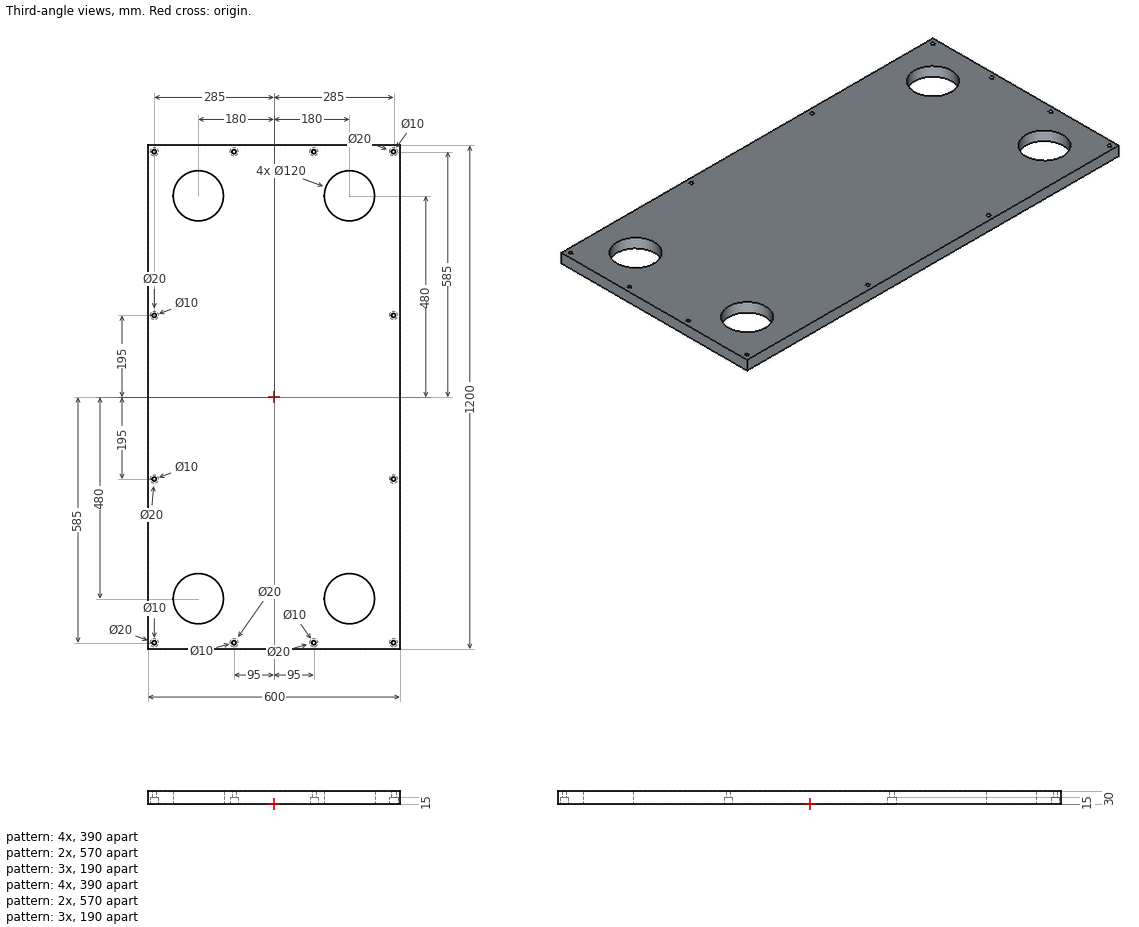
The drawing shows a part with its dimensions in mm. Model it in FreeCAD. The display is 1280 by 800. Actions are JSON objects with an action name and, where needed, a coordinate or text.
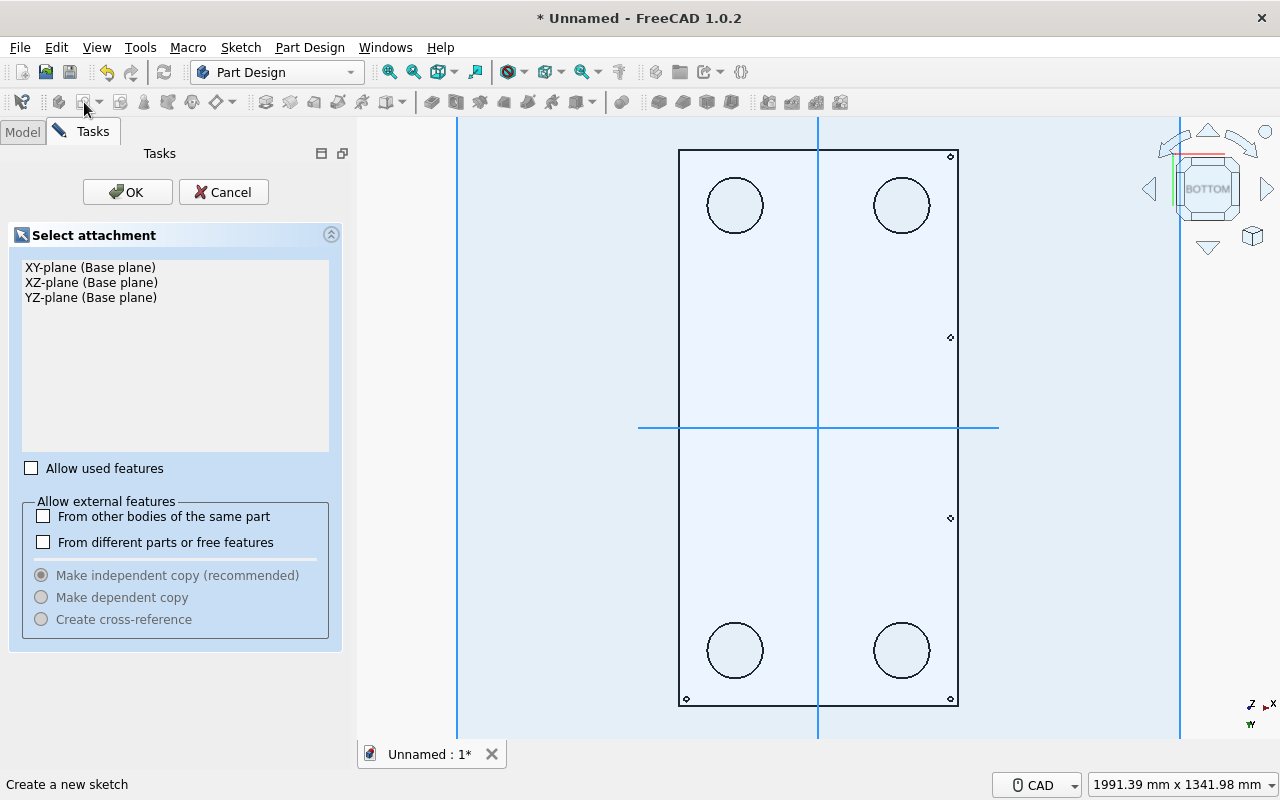
{"action": "left_click", "coordinate": [82, 268]}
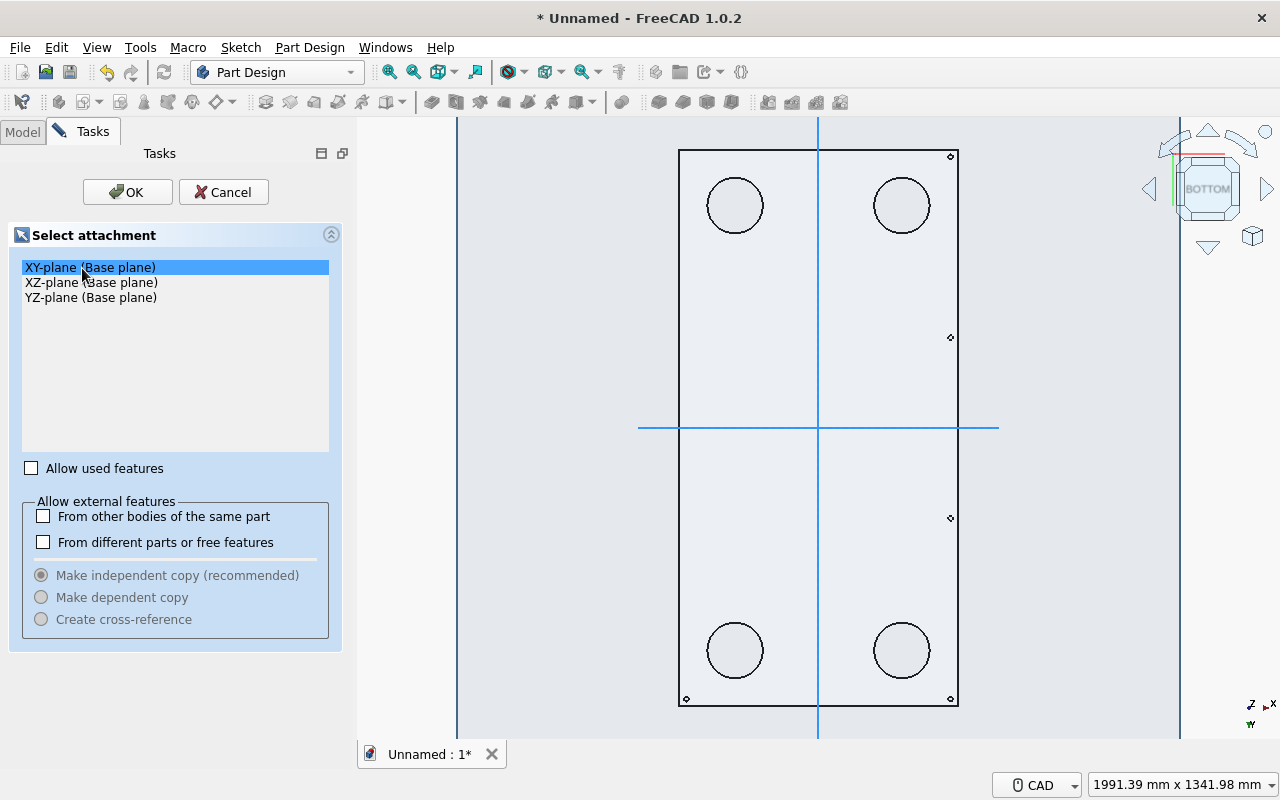
{"action": "left_click", "coordinate": [128, 192]}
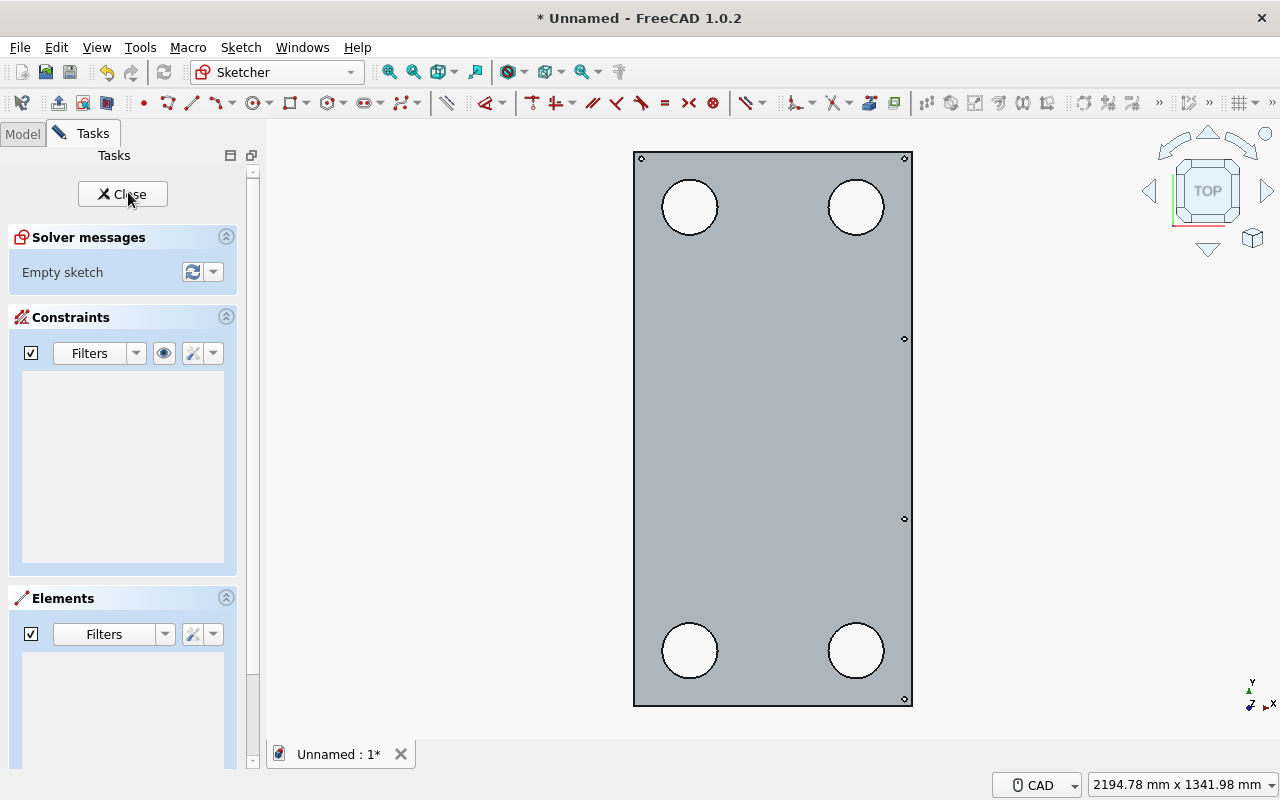
{"action": "left_click", "coordinate": [108, 104]}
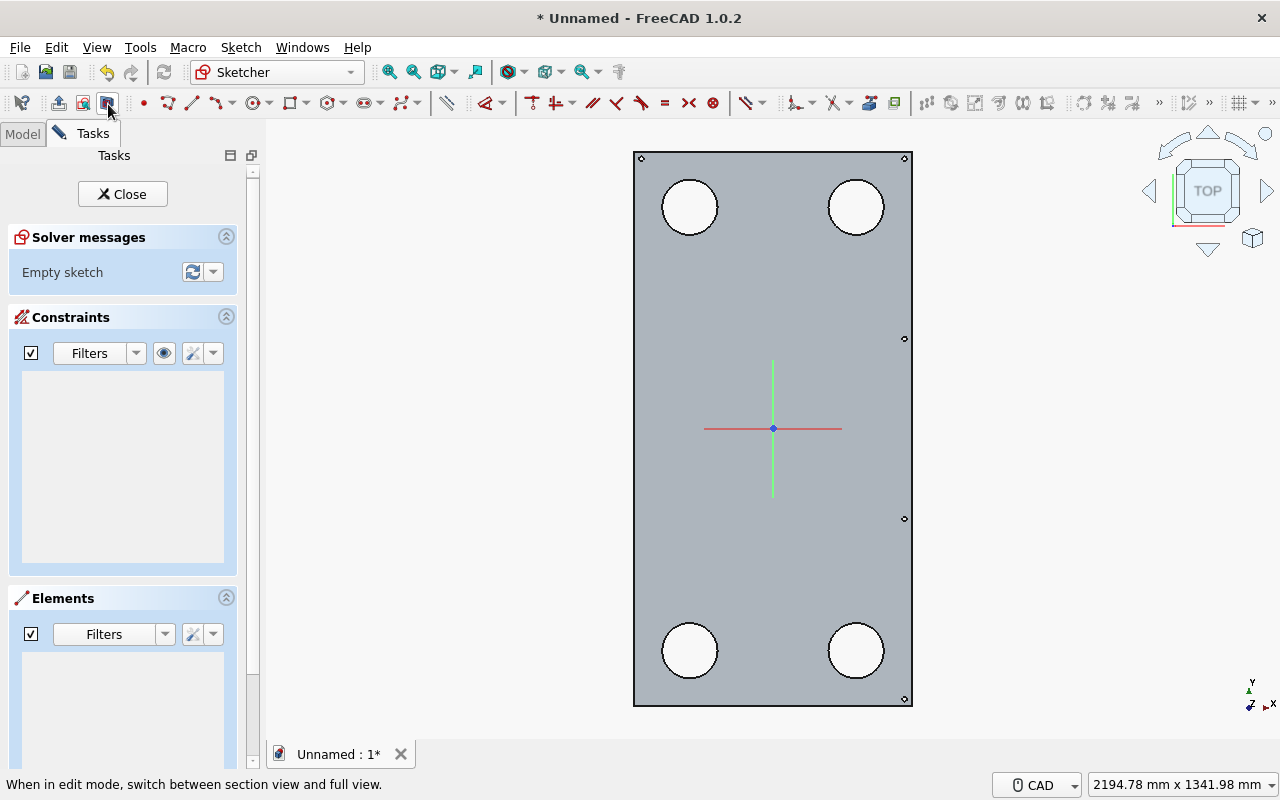
{"action": "scroll", "coordinate": [638, 334], "scroll_direction": "up", "scroll_amount": 15}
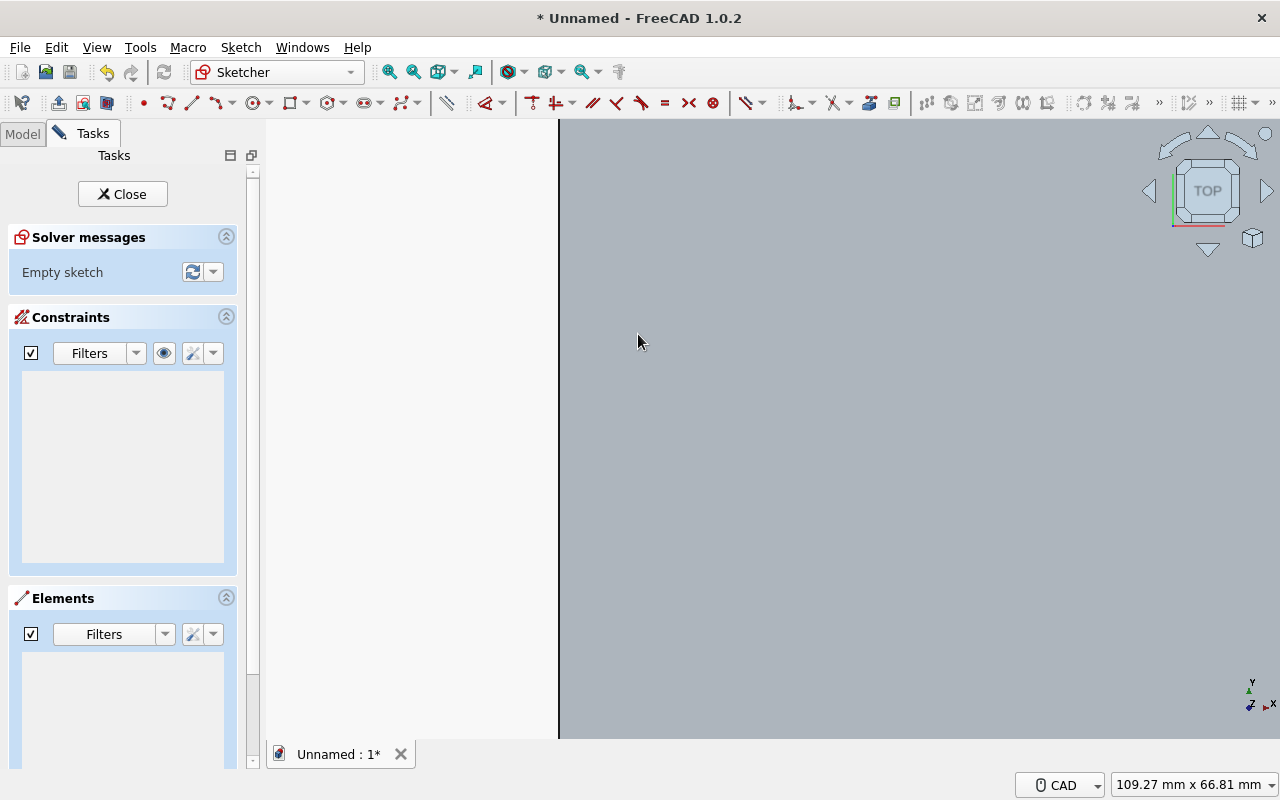
{"action": "scroll", "coordinate": [696, 425], "scroll_direction": "up", "scroll_amount": 7}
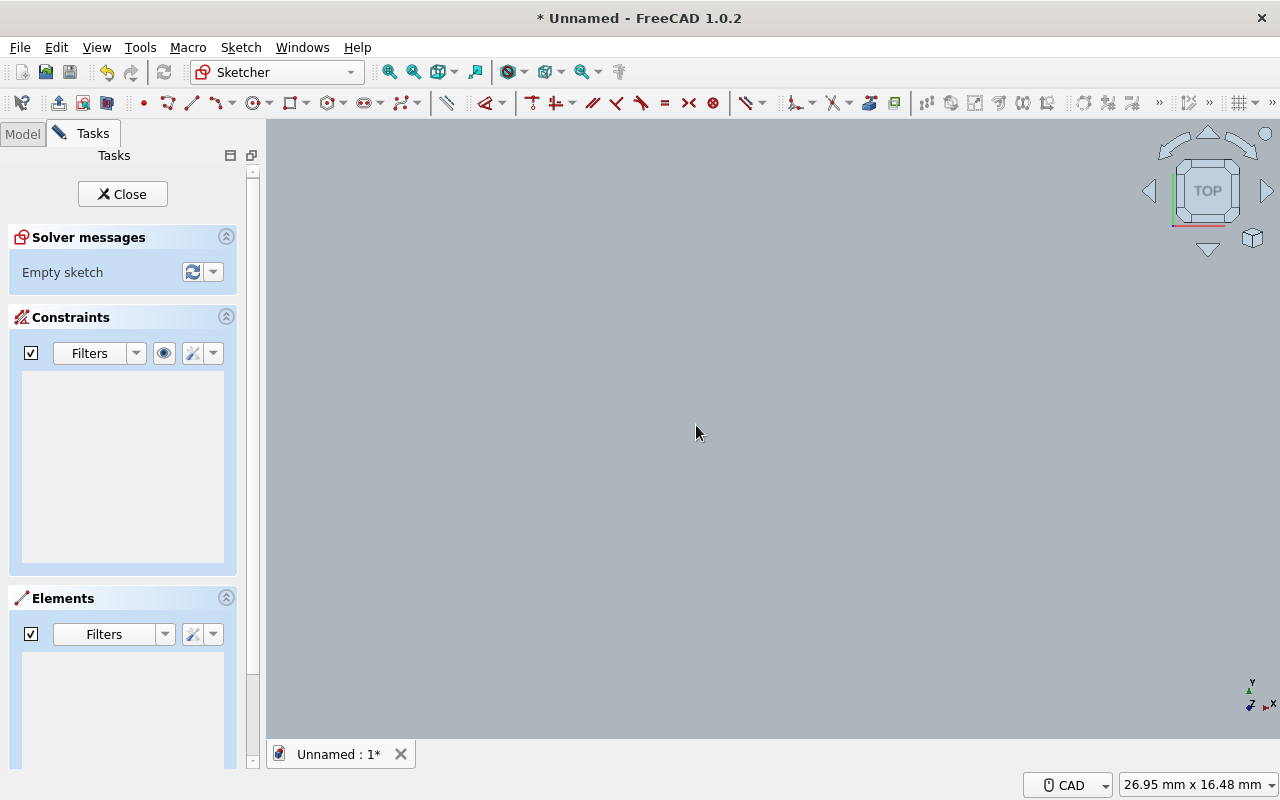
{"action": "left_click", "coordinate": [254, 104]}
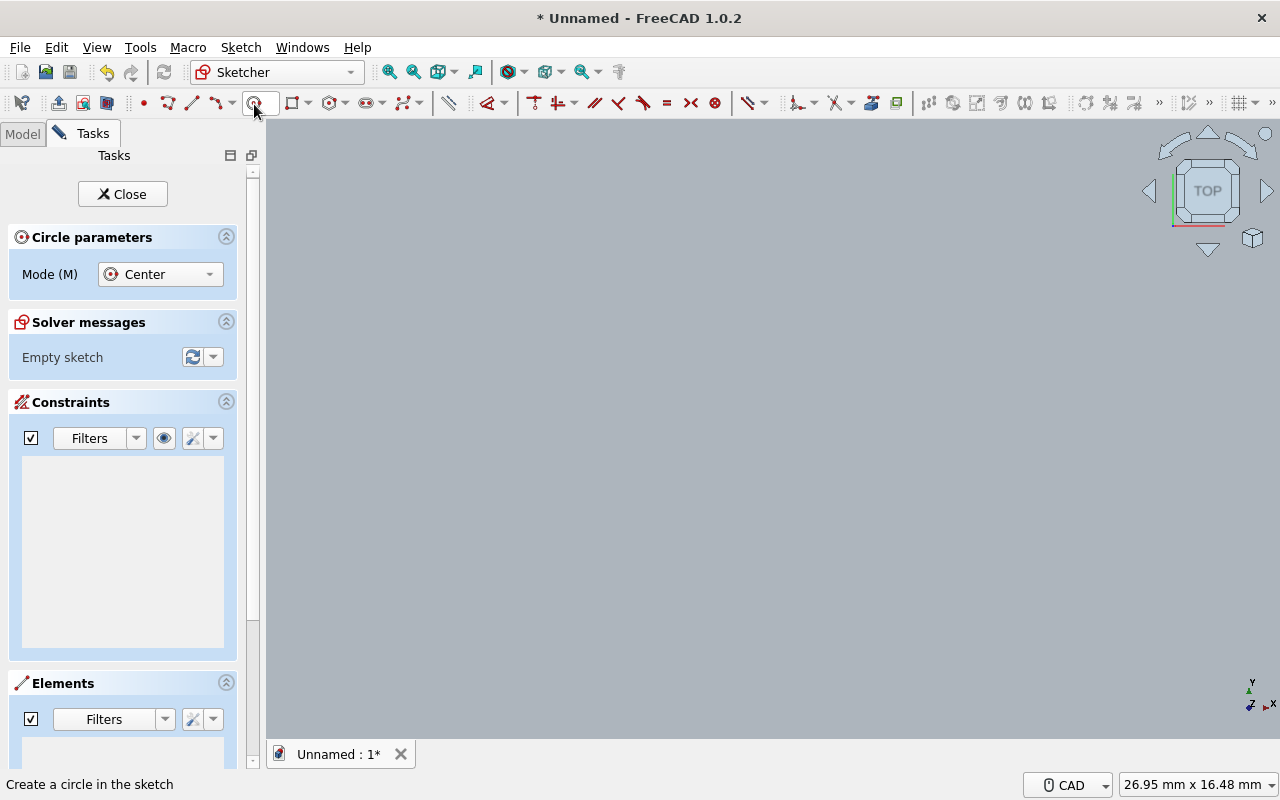
{"action": "left_click", "coordinate": [702, 427]}
{"action": "mouse_move", "coordinate": [835, 294]}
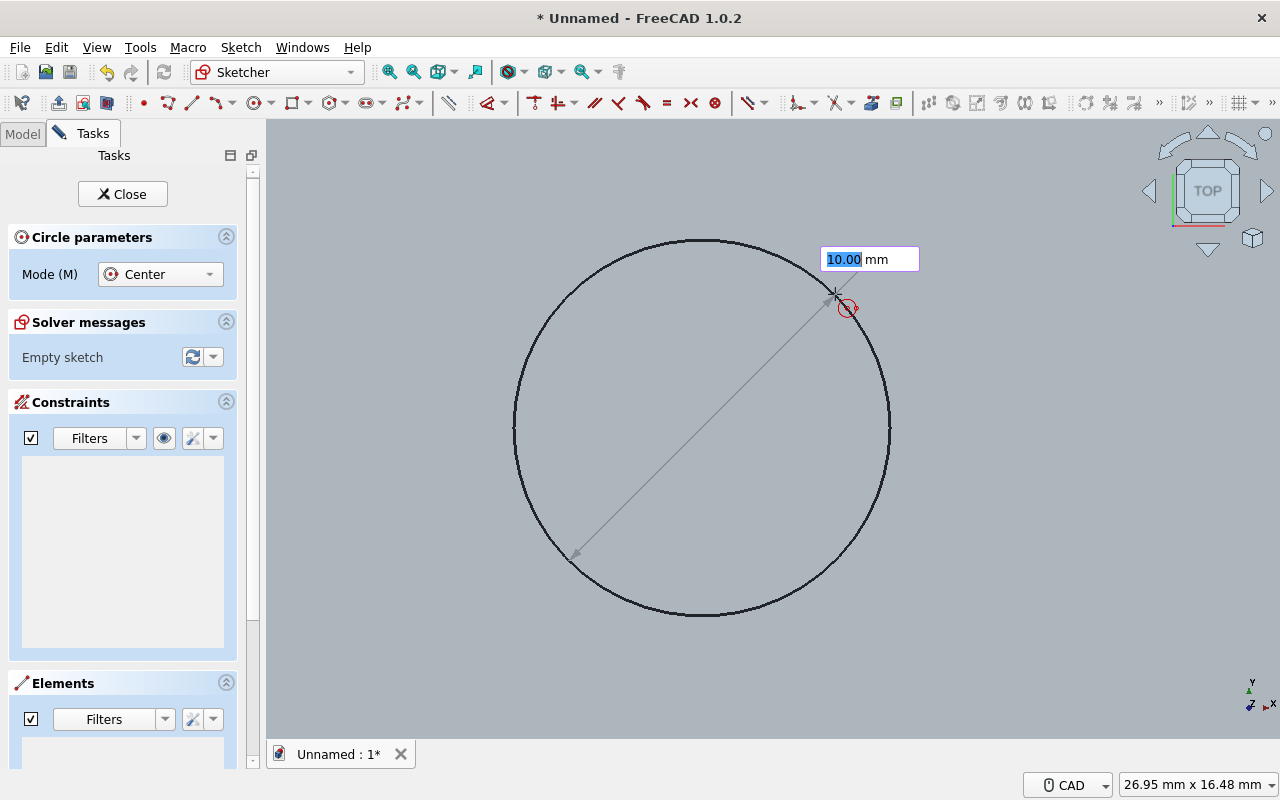
{"action": "type", "text": "10"}
{"action": "key", "text": "Return"}
{"action": "key", "text": "Escape"}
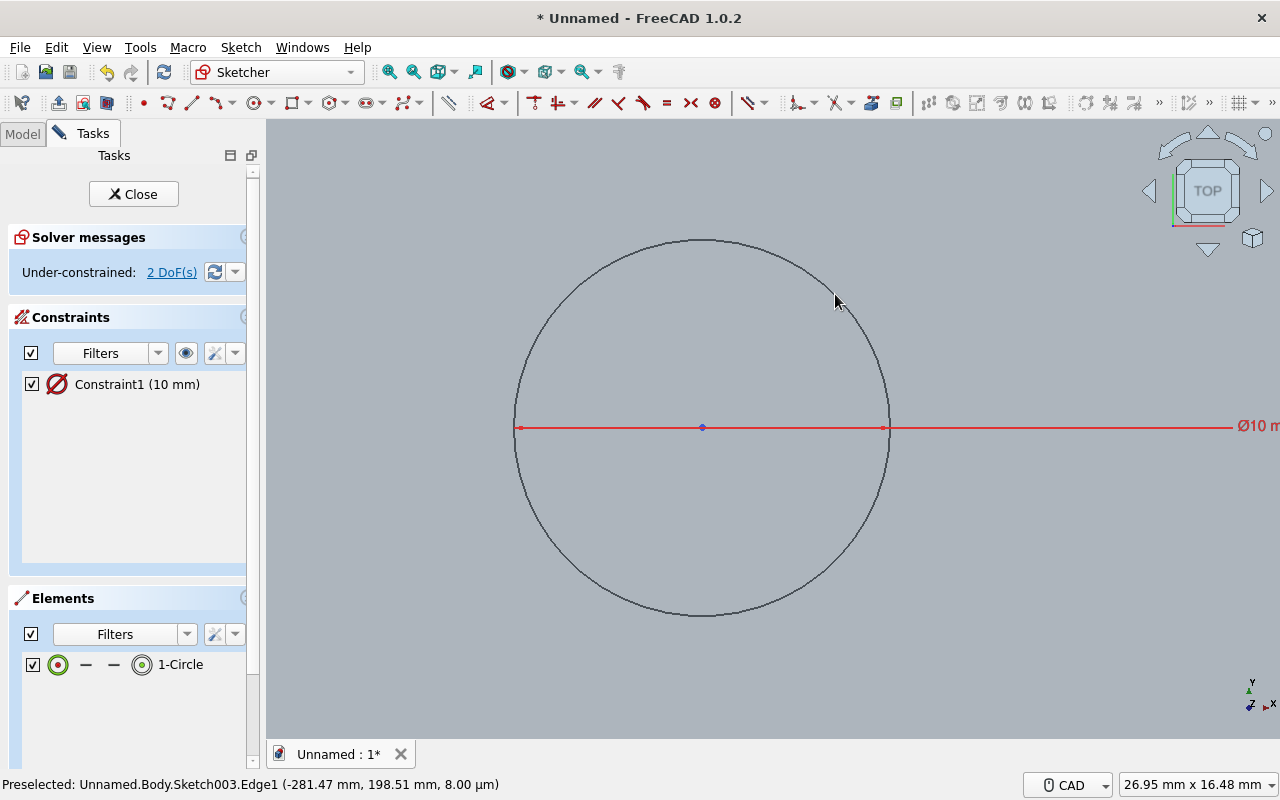
{"action": "left_click", "coordinate": [488, 104]}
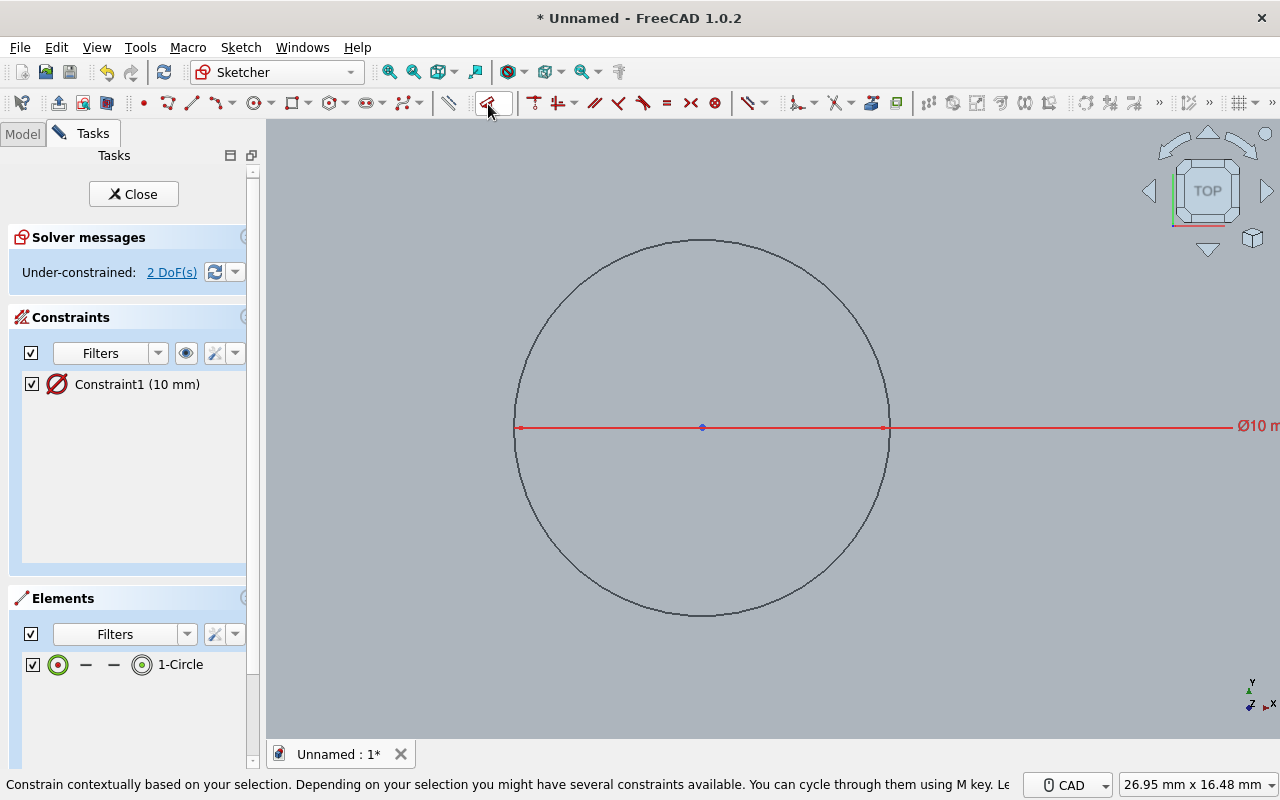
{"action": "left_click", "coordinate": [702, 428]}
{"action": "left_click", "coordinate": [909, 394]}